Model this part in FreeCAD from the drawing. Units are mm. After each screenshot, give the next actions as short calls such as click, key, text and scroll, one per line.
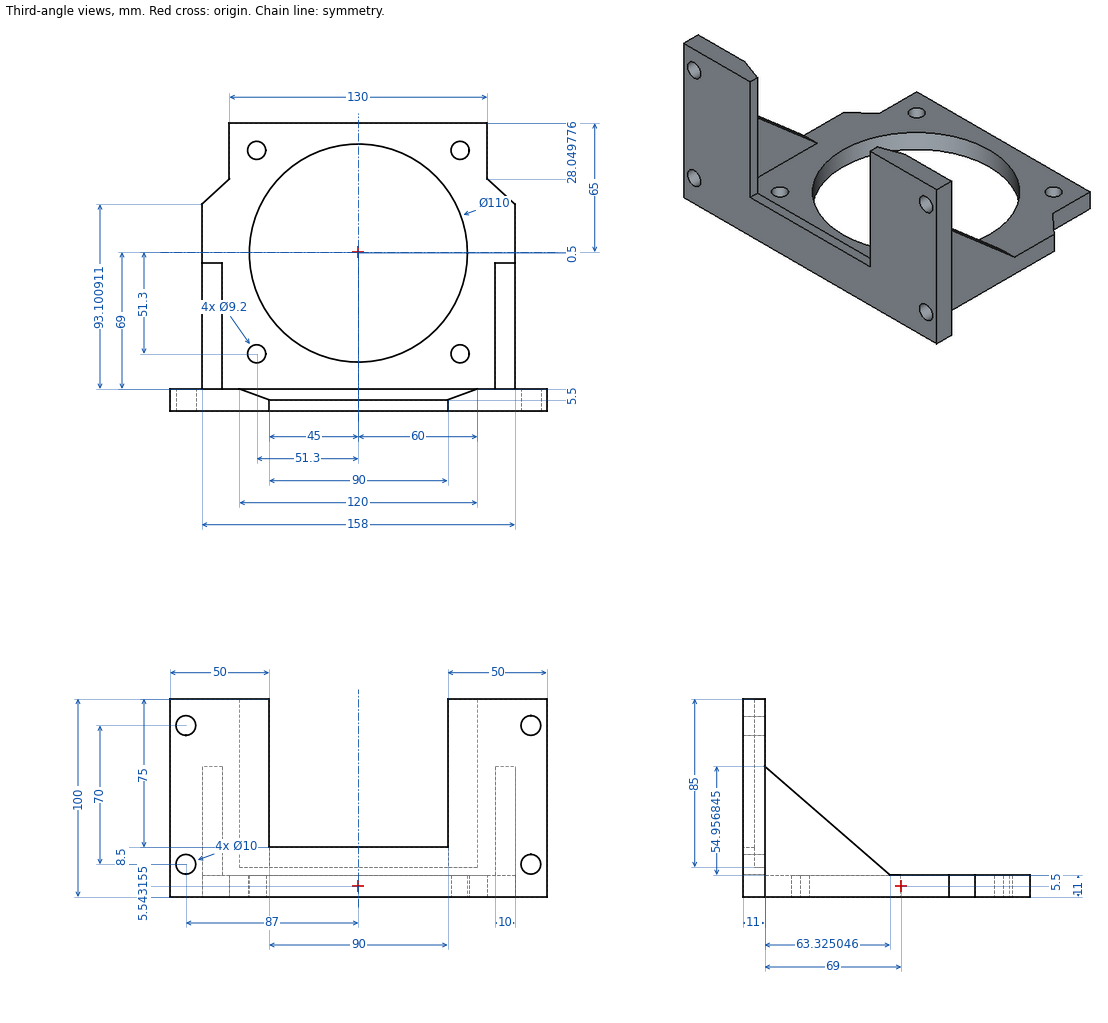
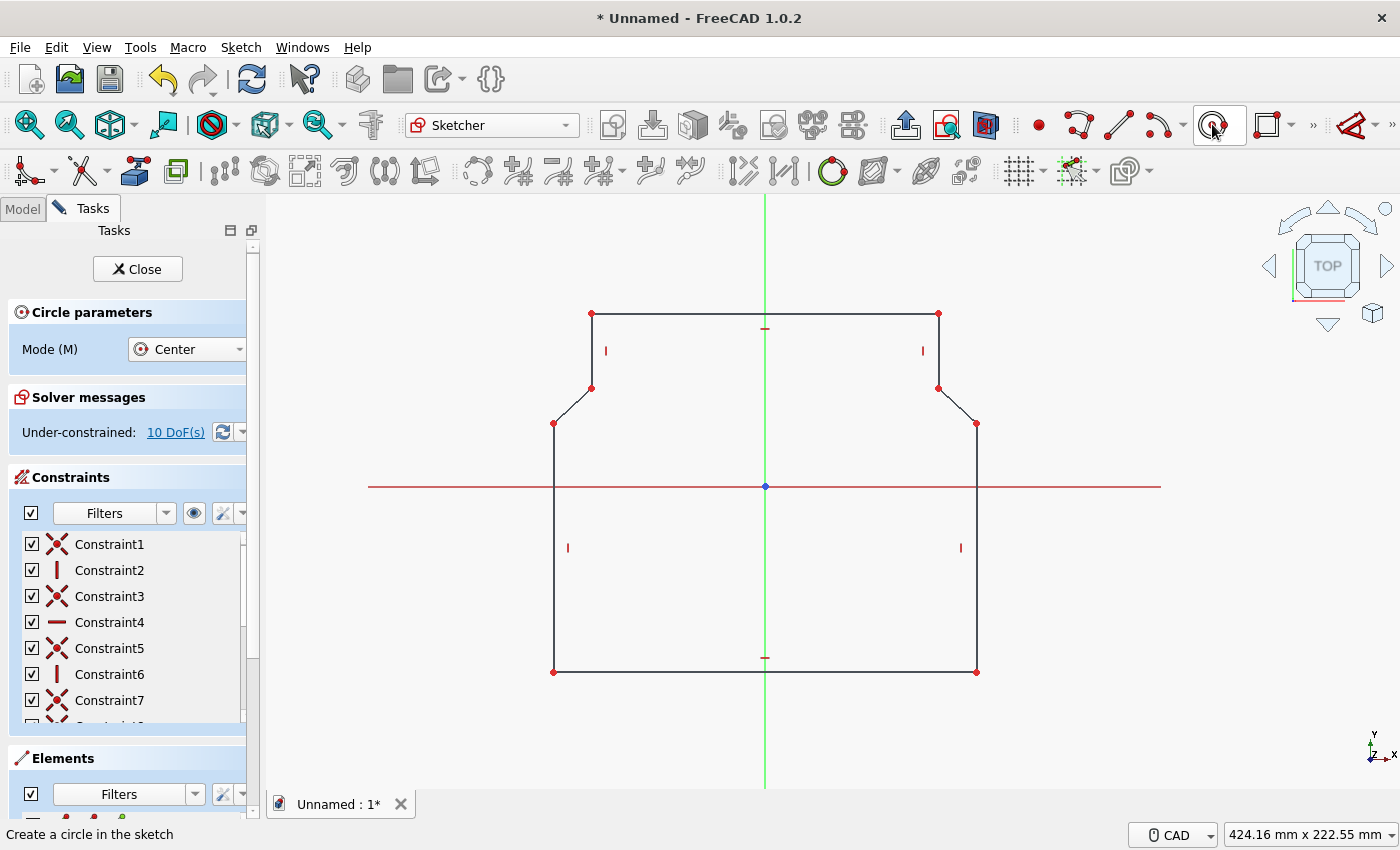
scroll(628, 624, up, 4)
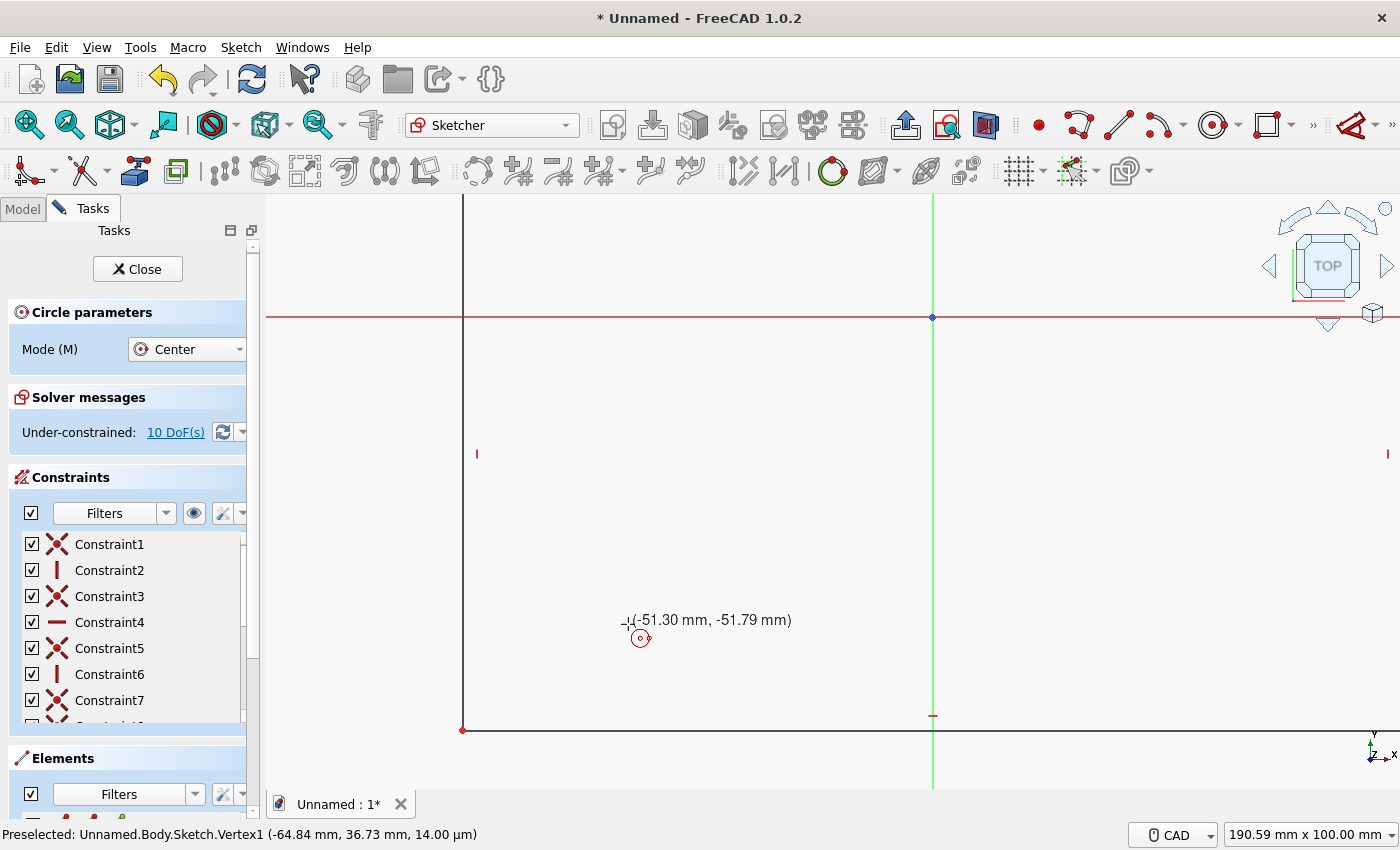
click(628, 622)
move(647, 603)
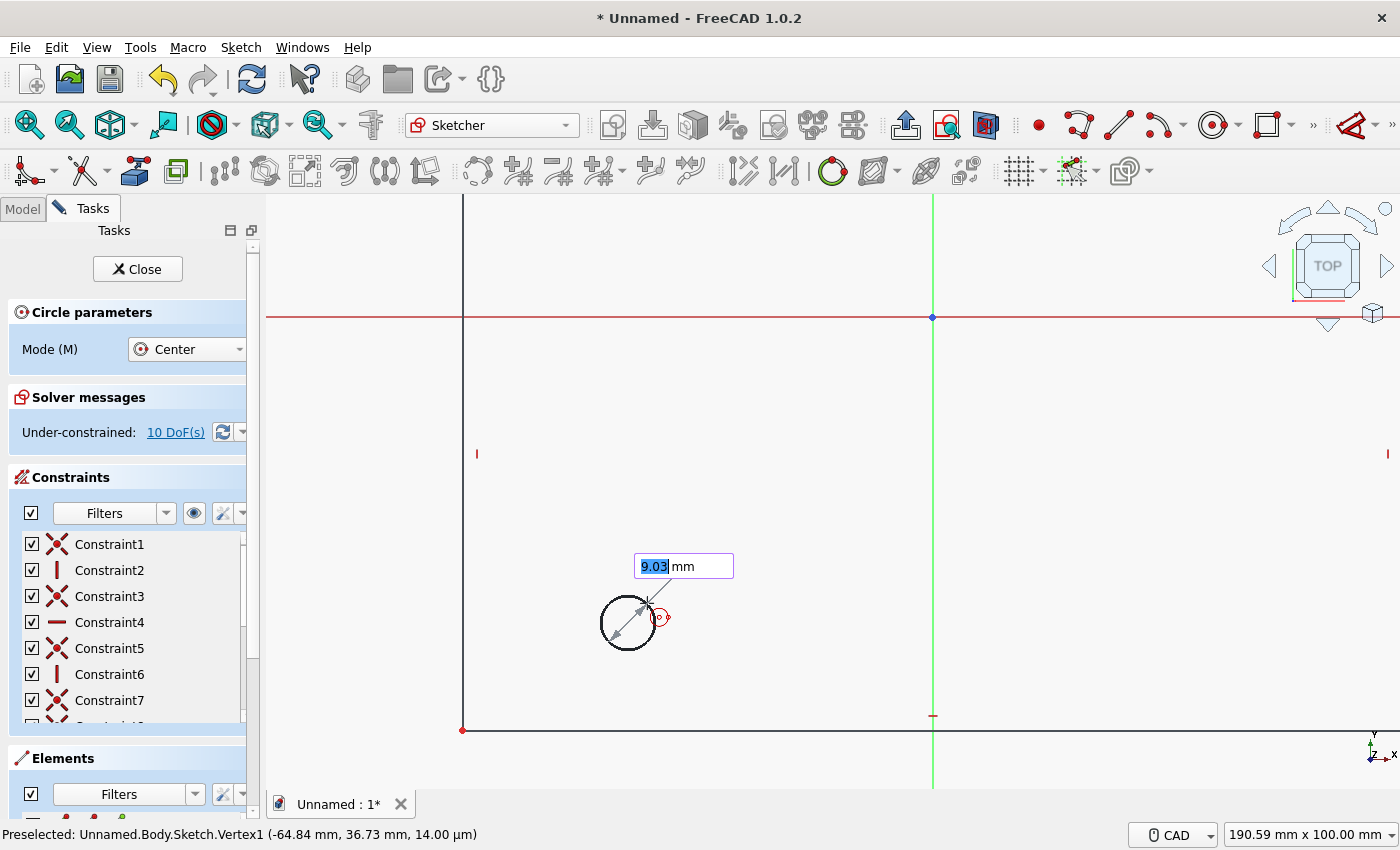
text(9.2)
key(Return)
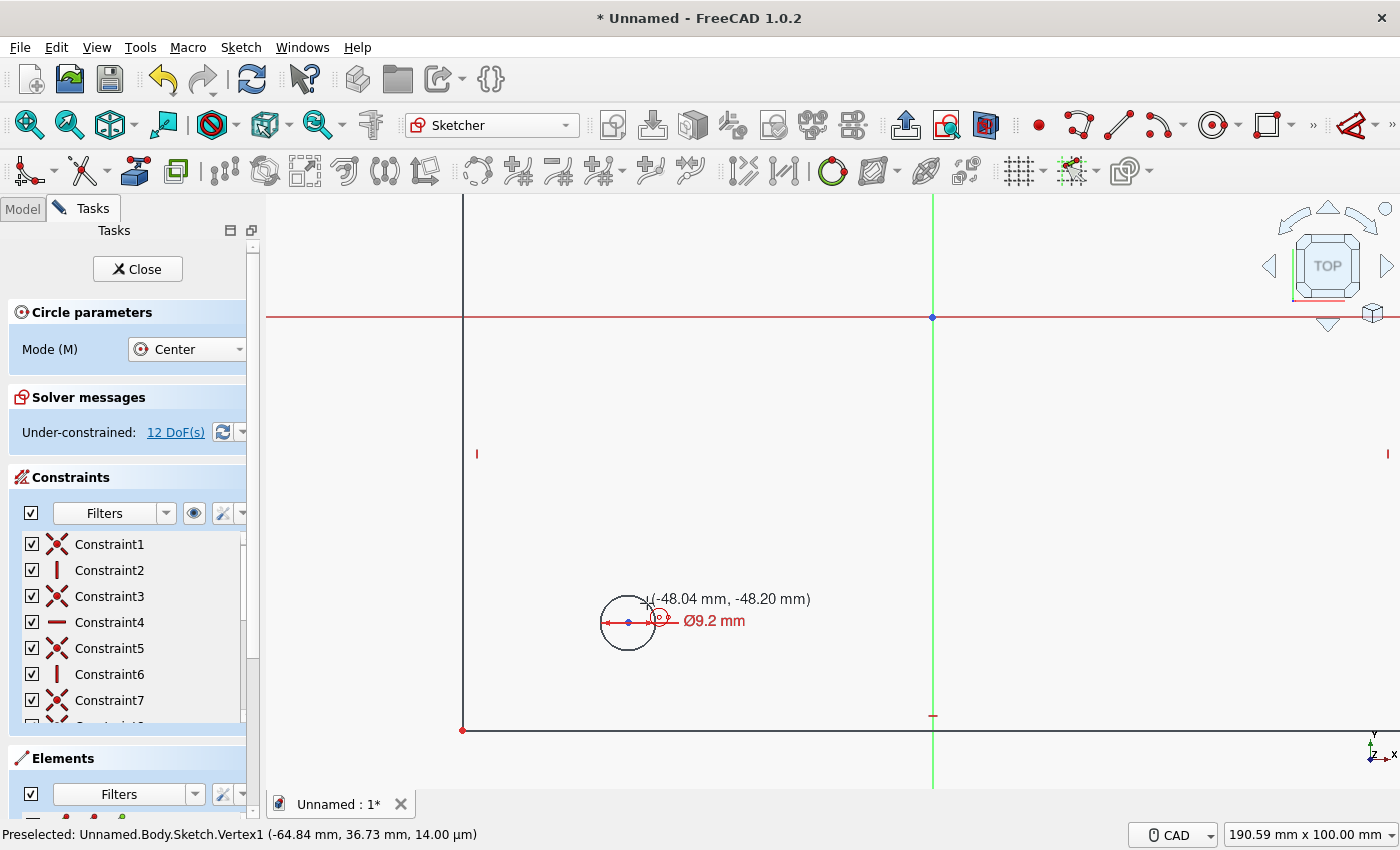
scroll(933, 320, up, 9)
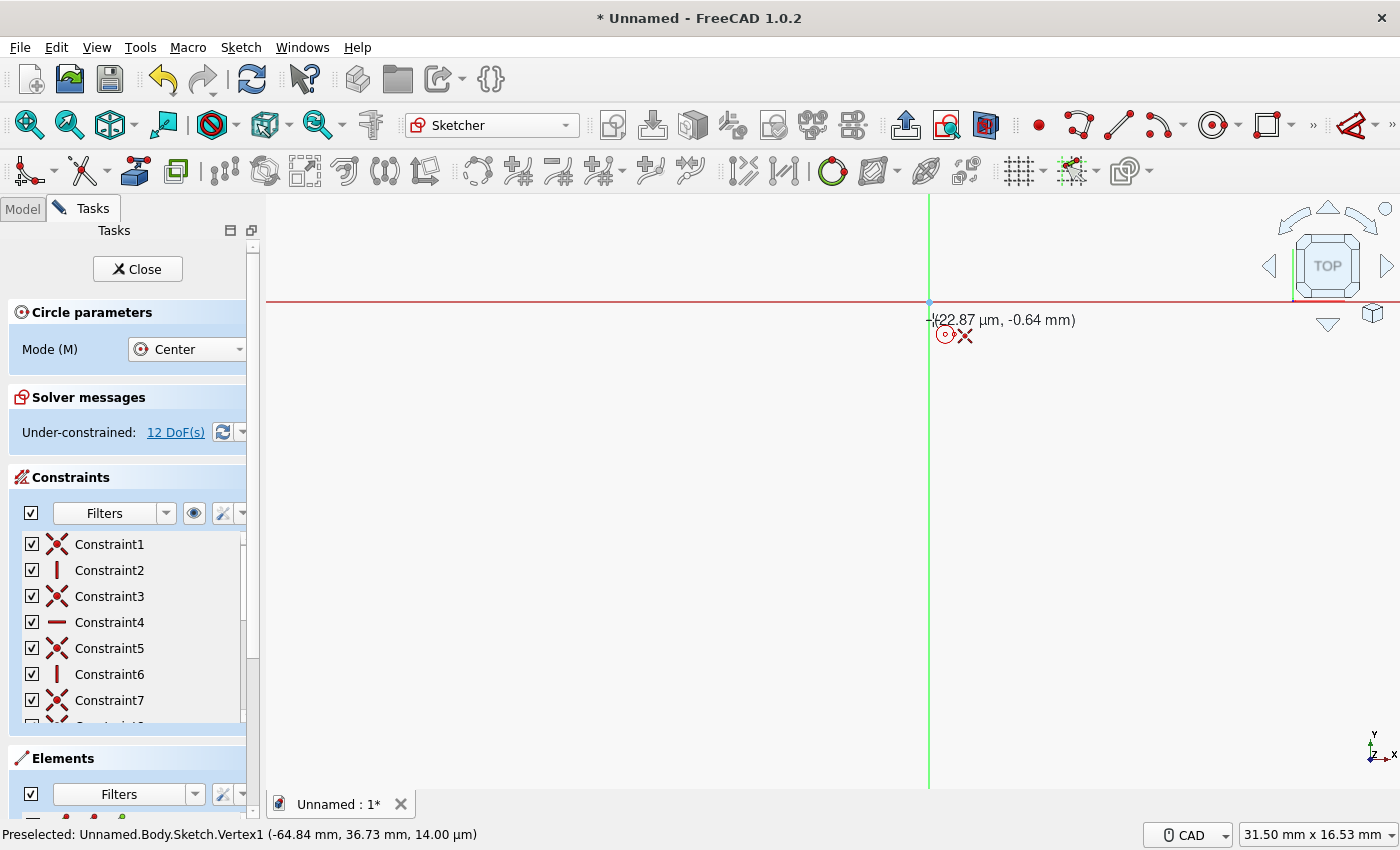
click(929, 320)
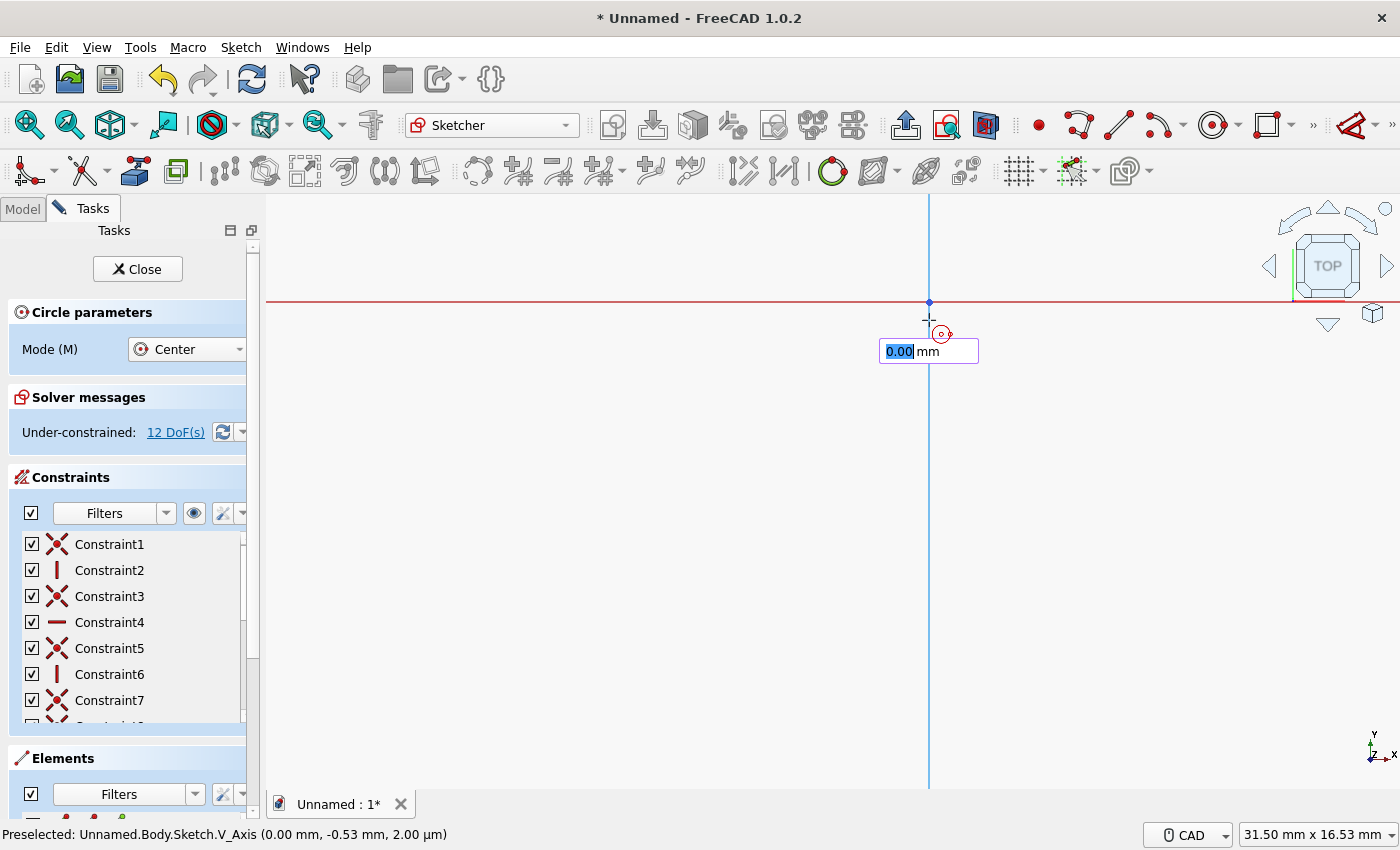
scroll(751, 501, down, 13)
move(869, 384)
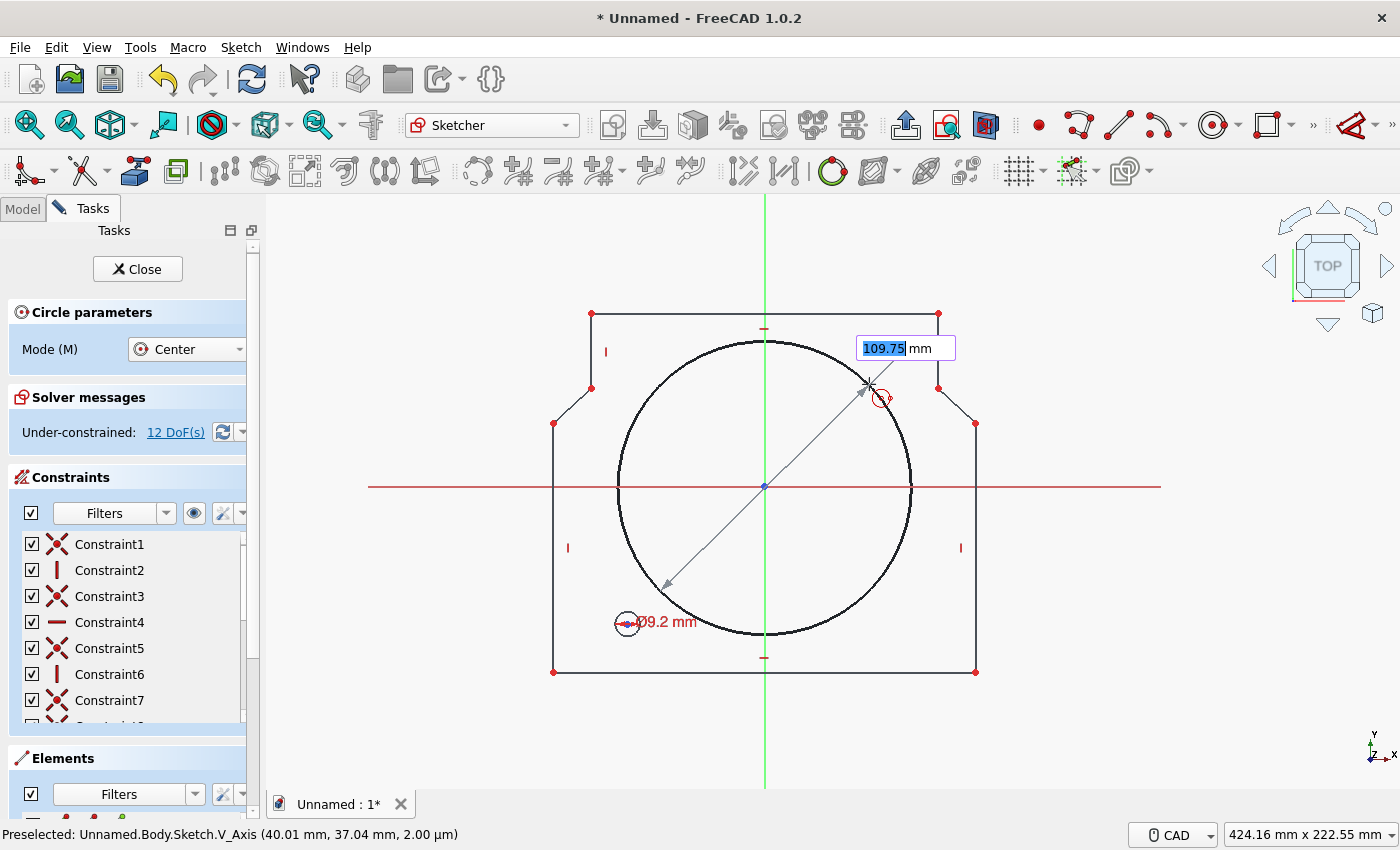
text(110)
key(Return)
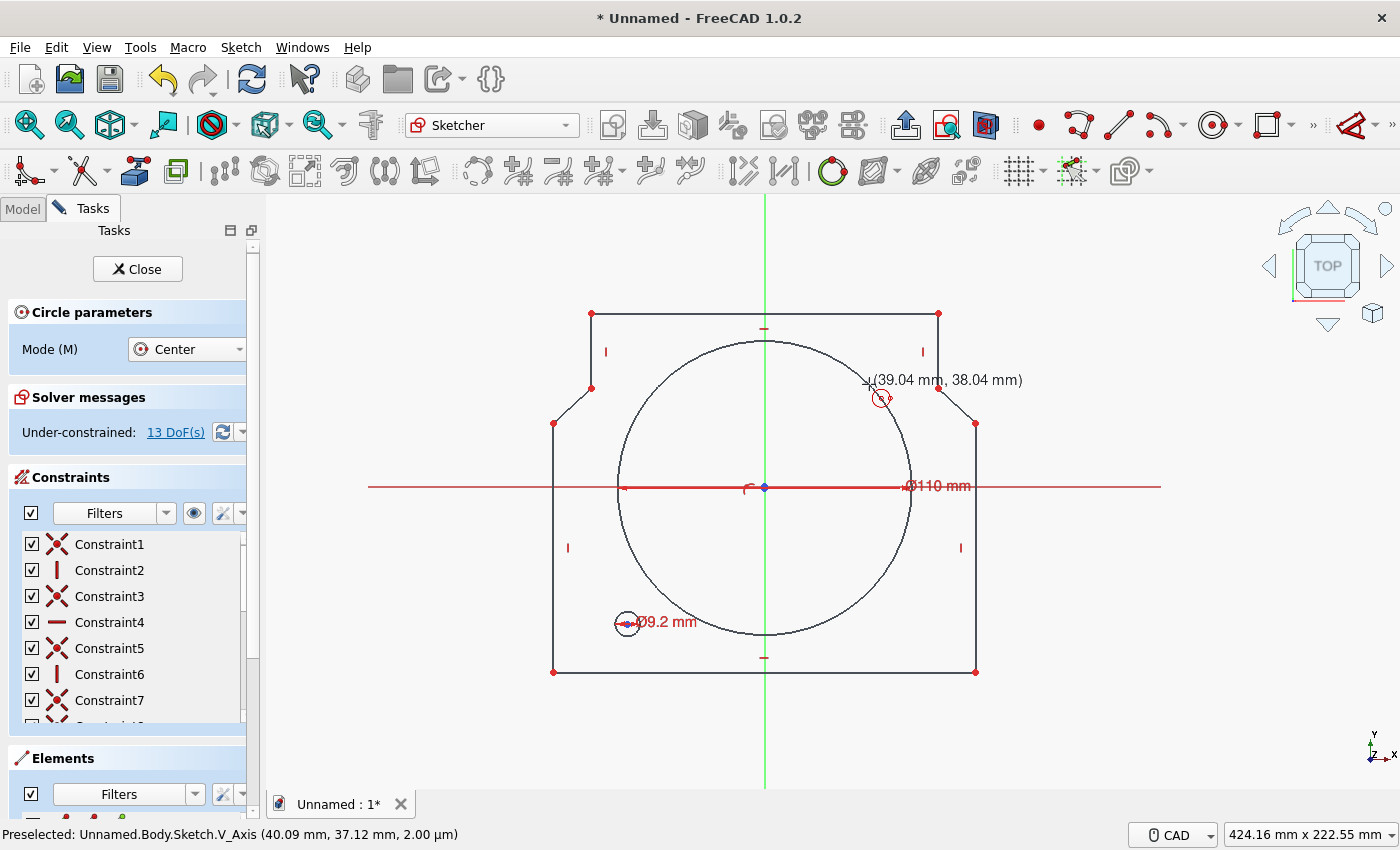
scroll(902, 624, up, 4)